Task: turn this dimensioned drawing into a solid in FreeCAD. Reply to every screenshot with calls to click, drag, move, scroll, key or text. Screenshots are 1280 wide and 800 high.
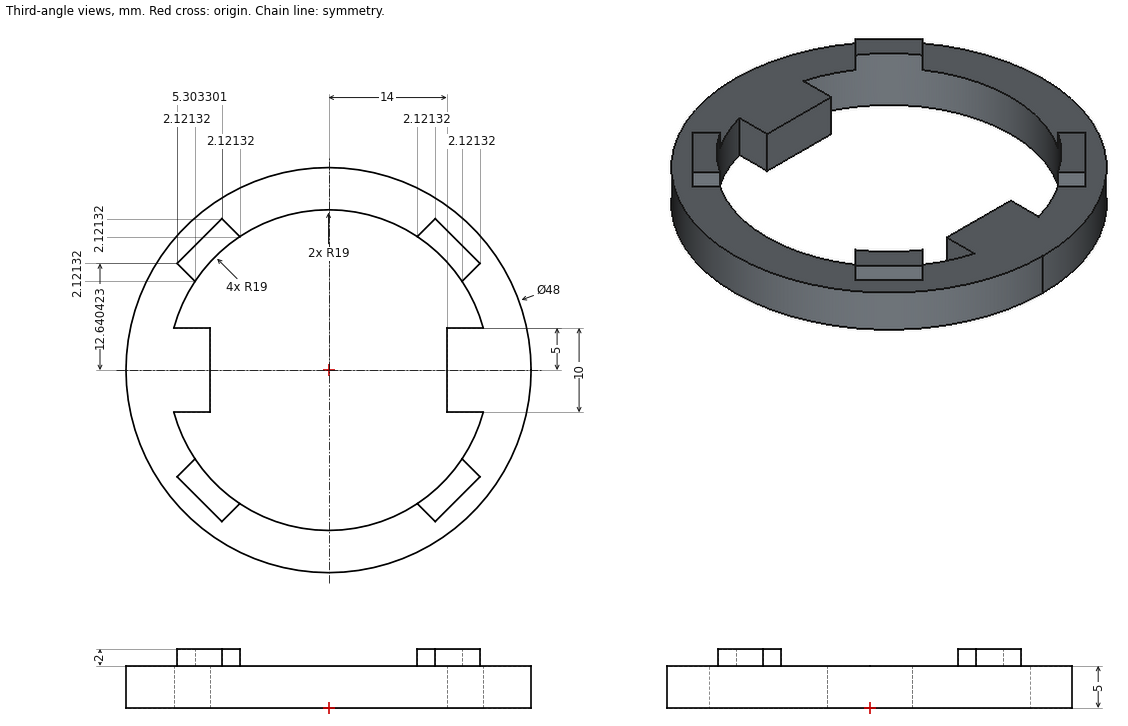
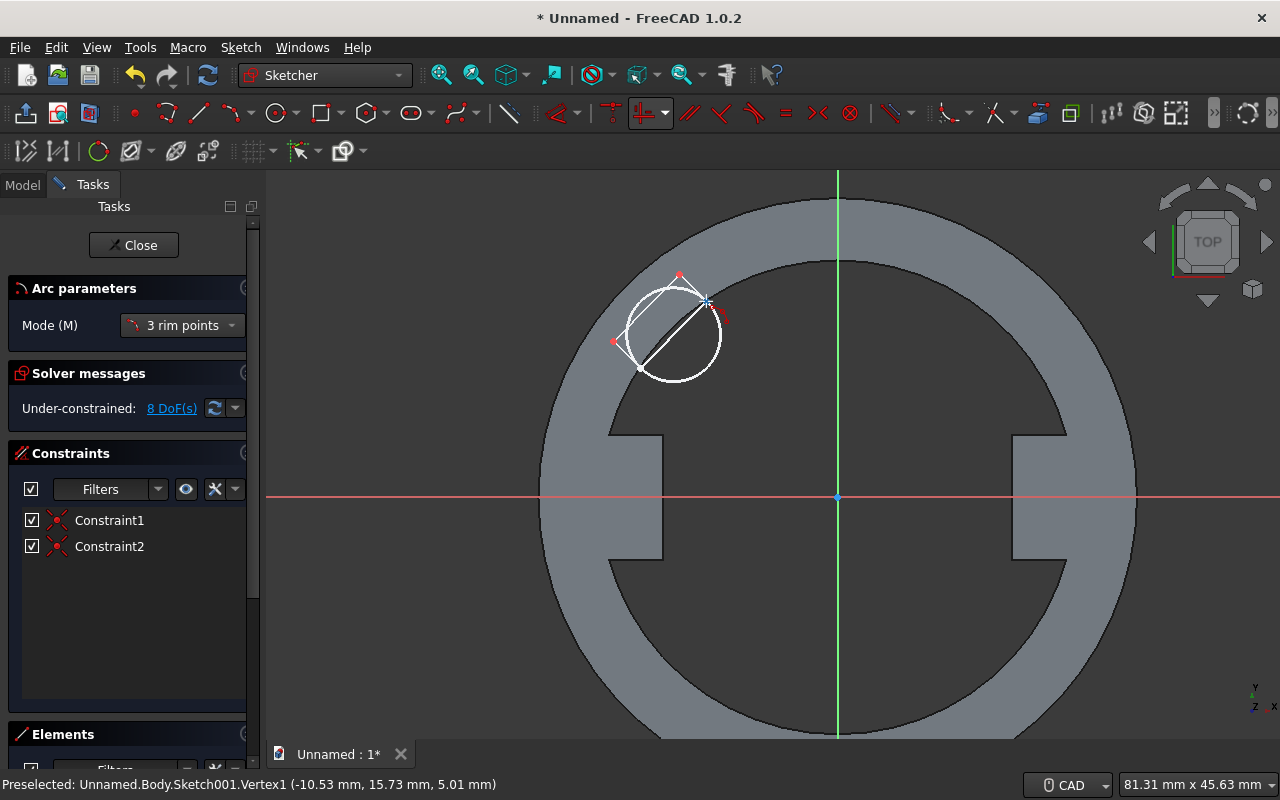
scroll(670, 330, up, 7)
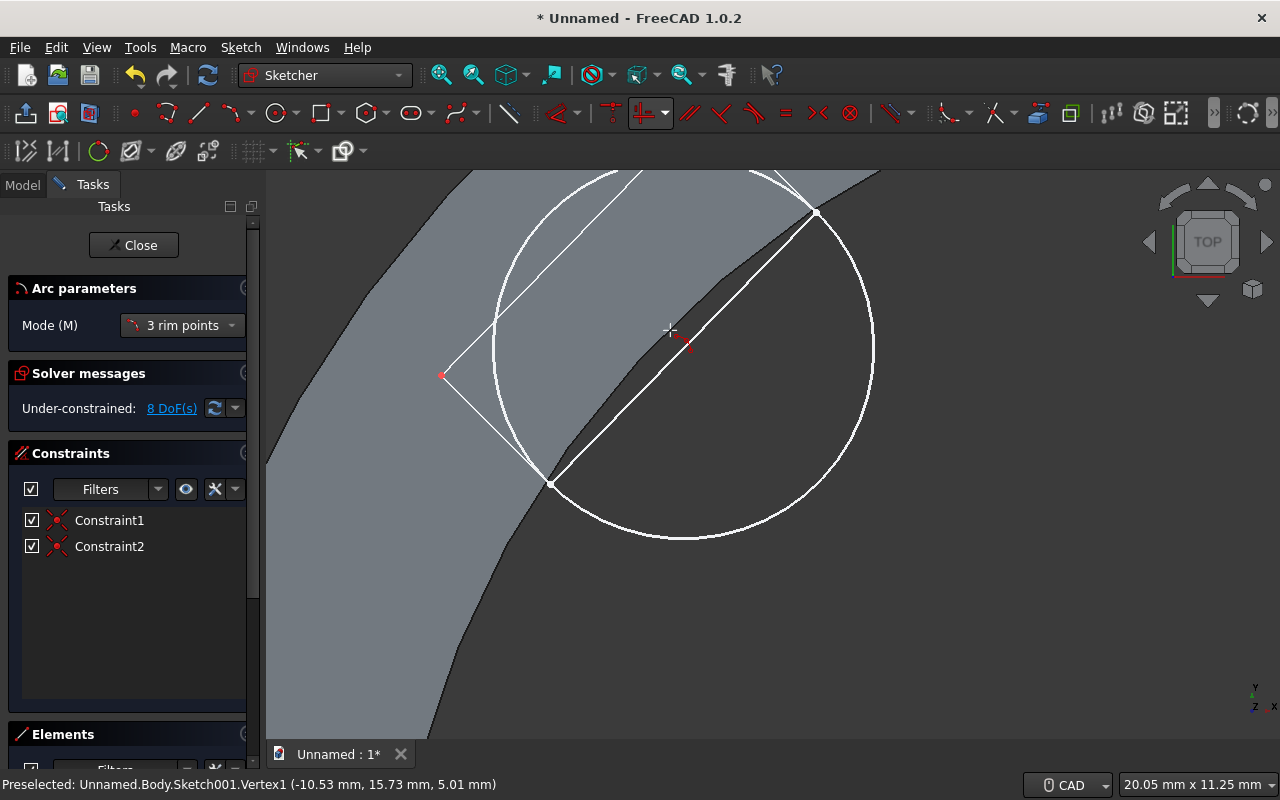
click(670, 328)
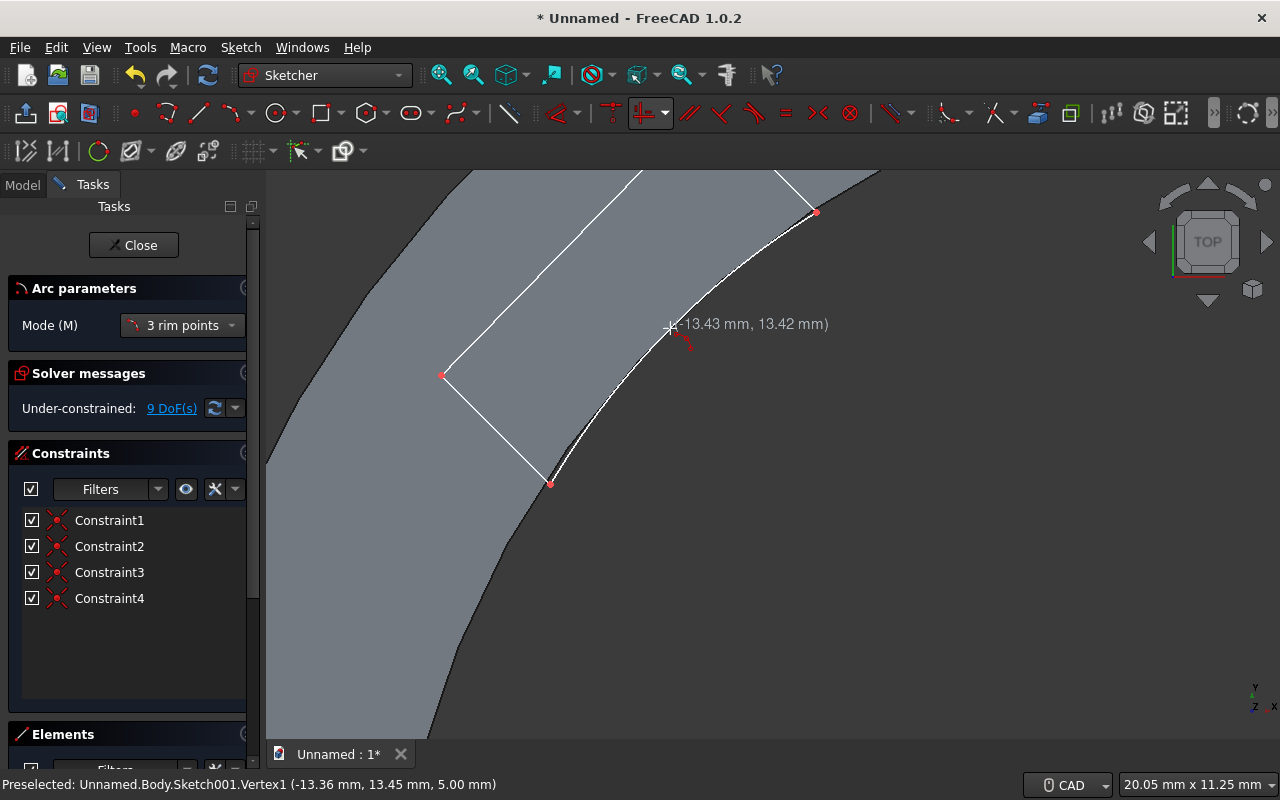
key(g)
key(m)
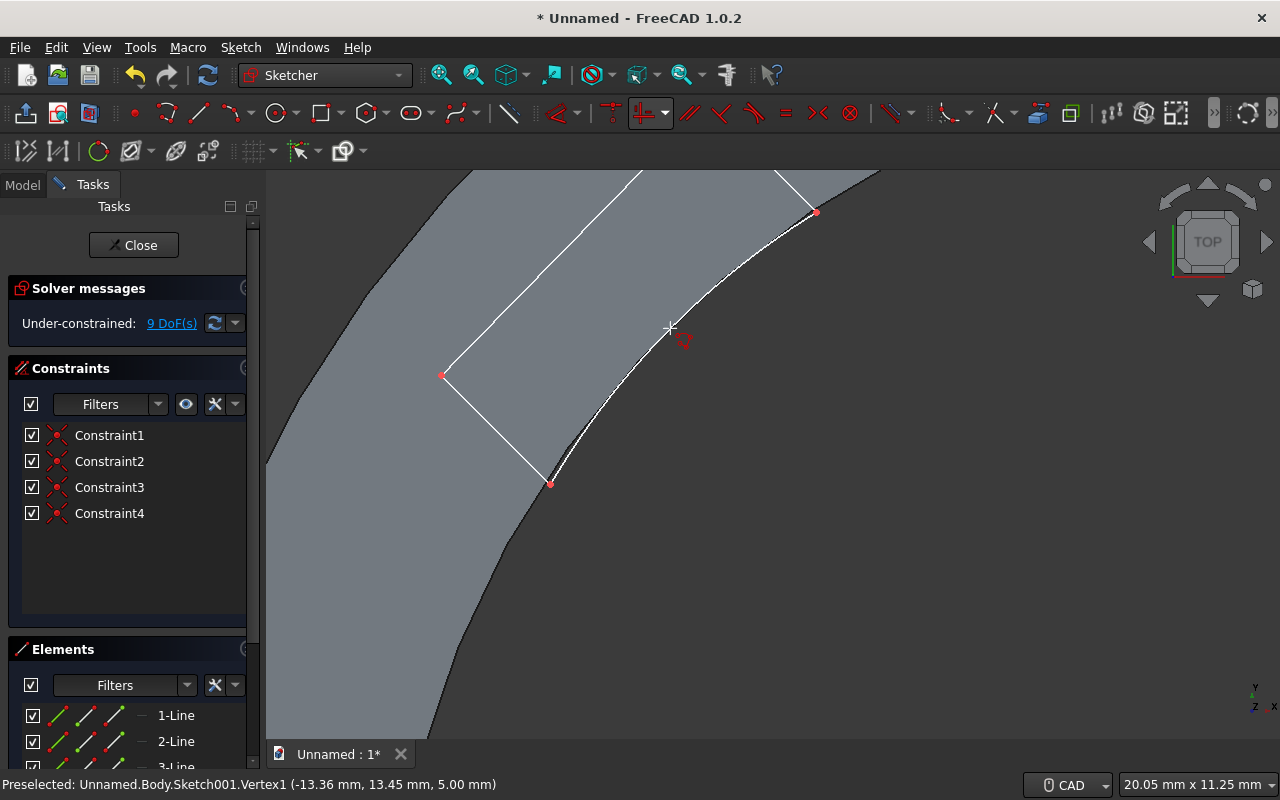
scroll(541, 315, down, 8)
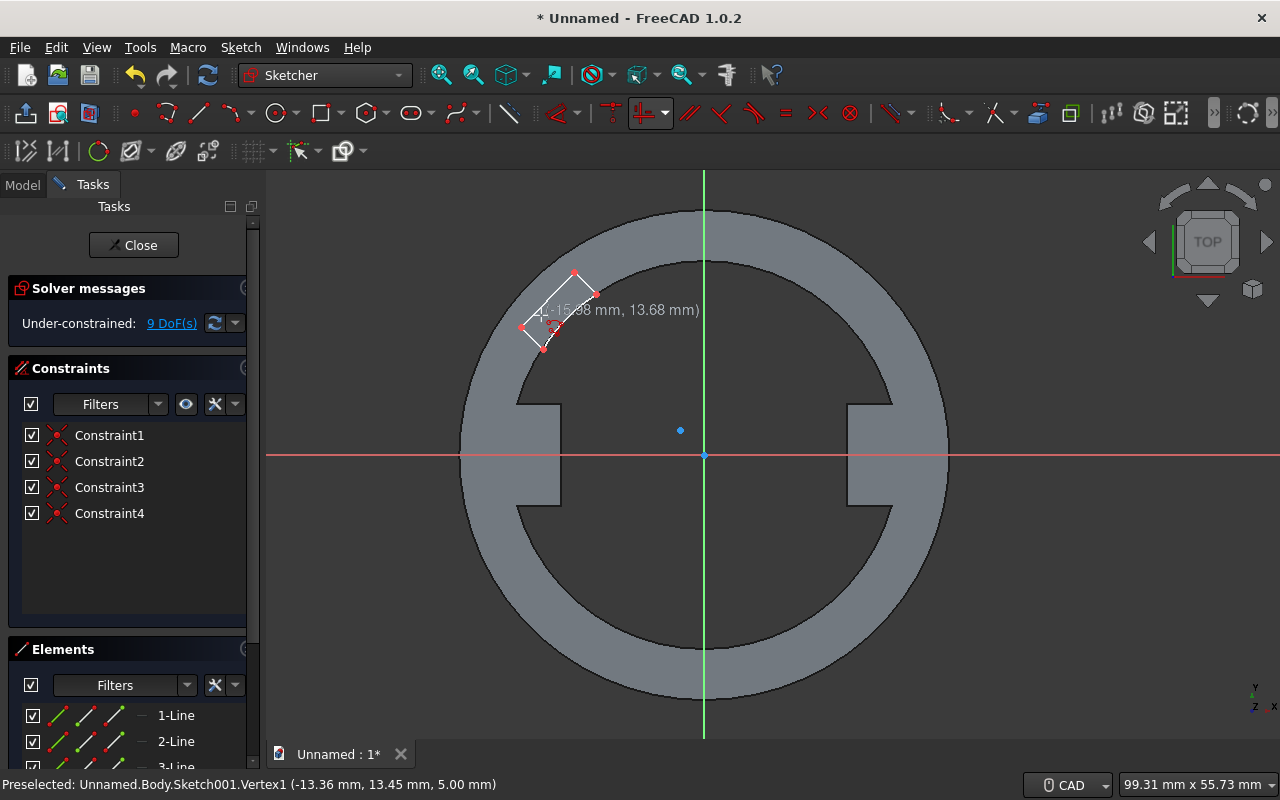
click(866, 348)
click(888, 326)
click(833, 272)
click(812, 294)
right_click(812, 294)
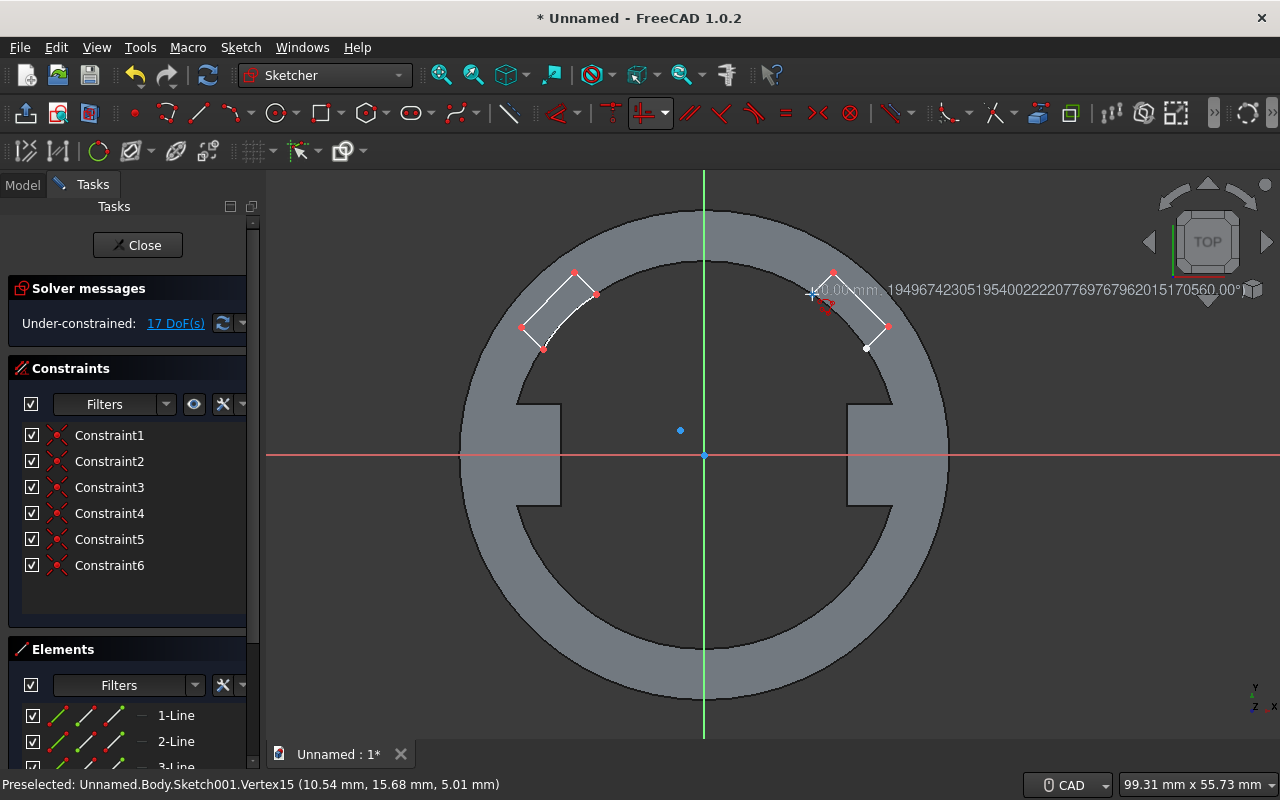
key(g)
key(3)
key(a)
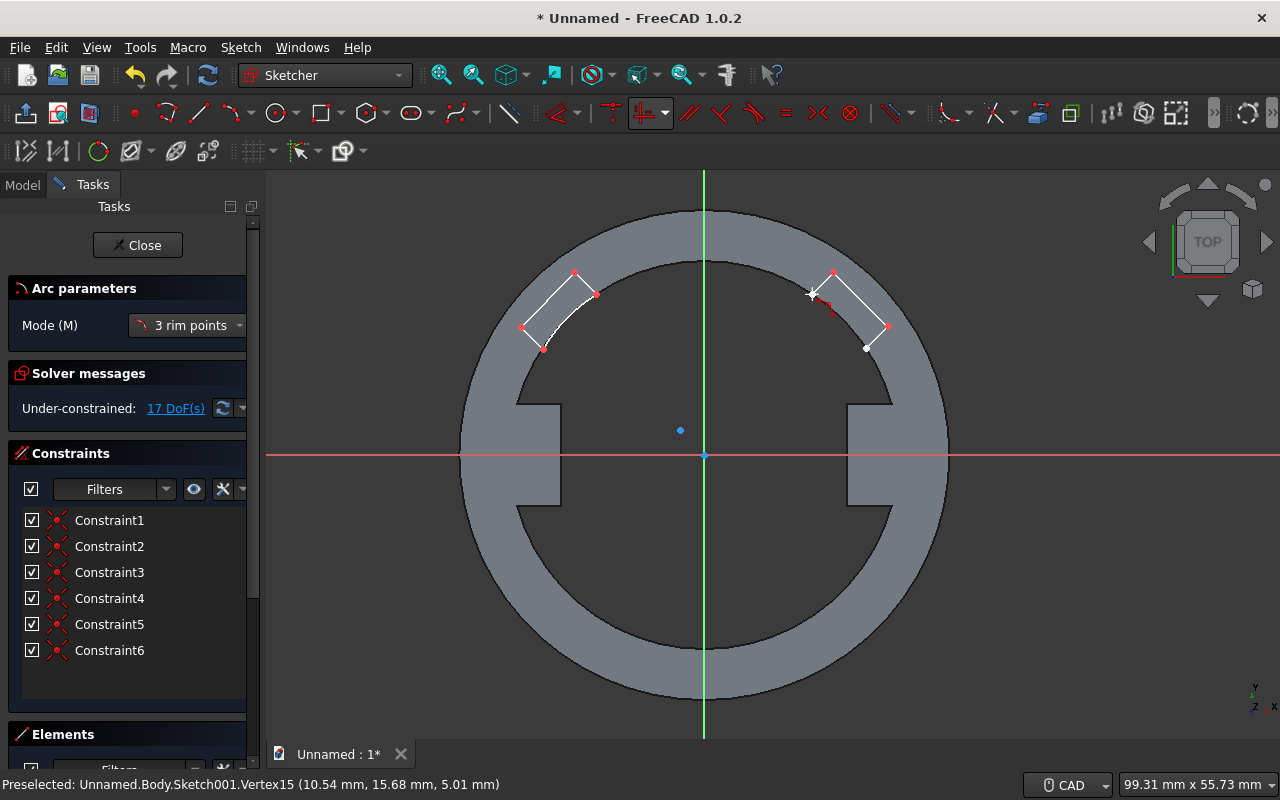
click(812, 295)
click(866, 349)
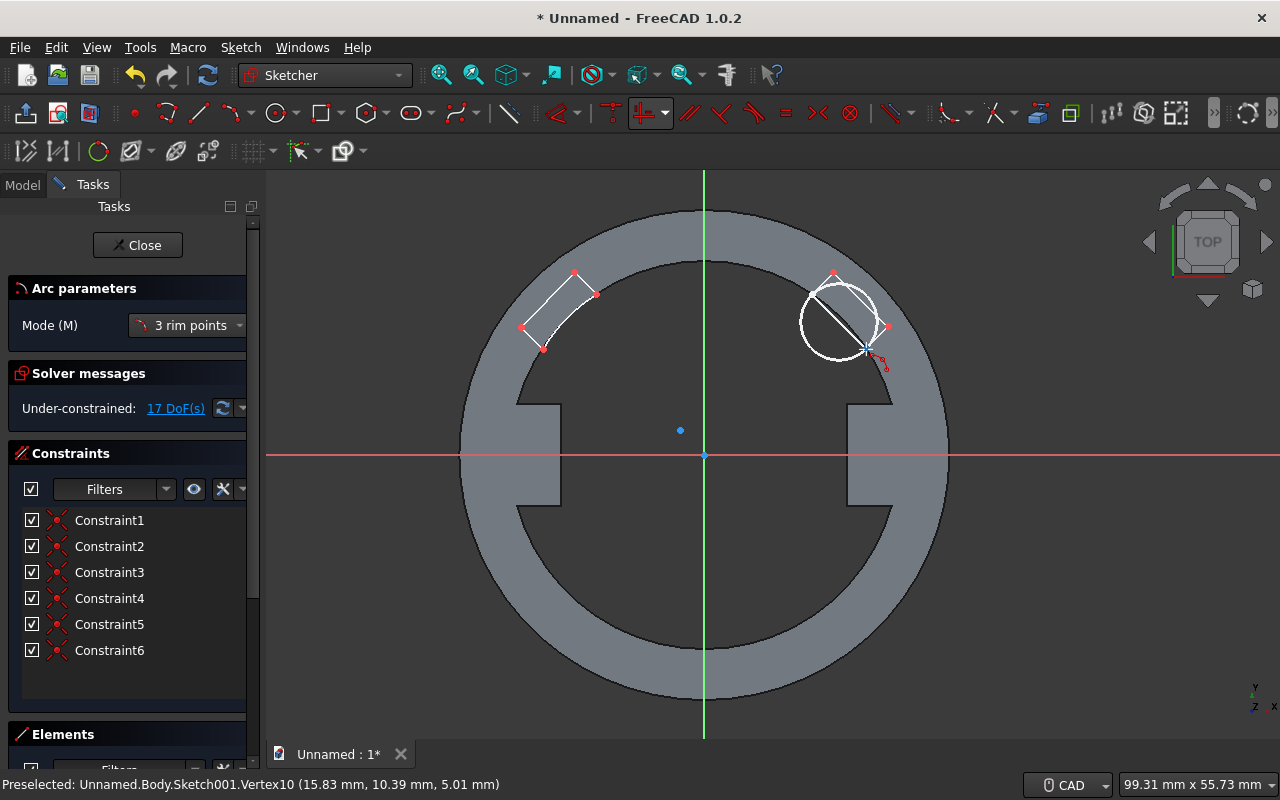
scroll(842, 318, up, 8)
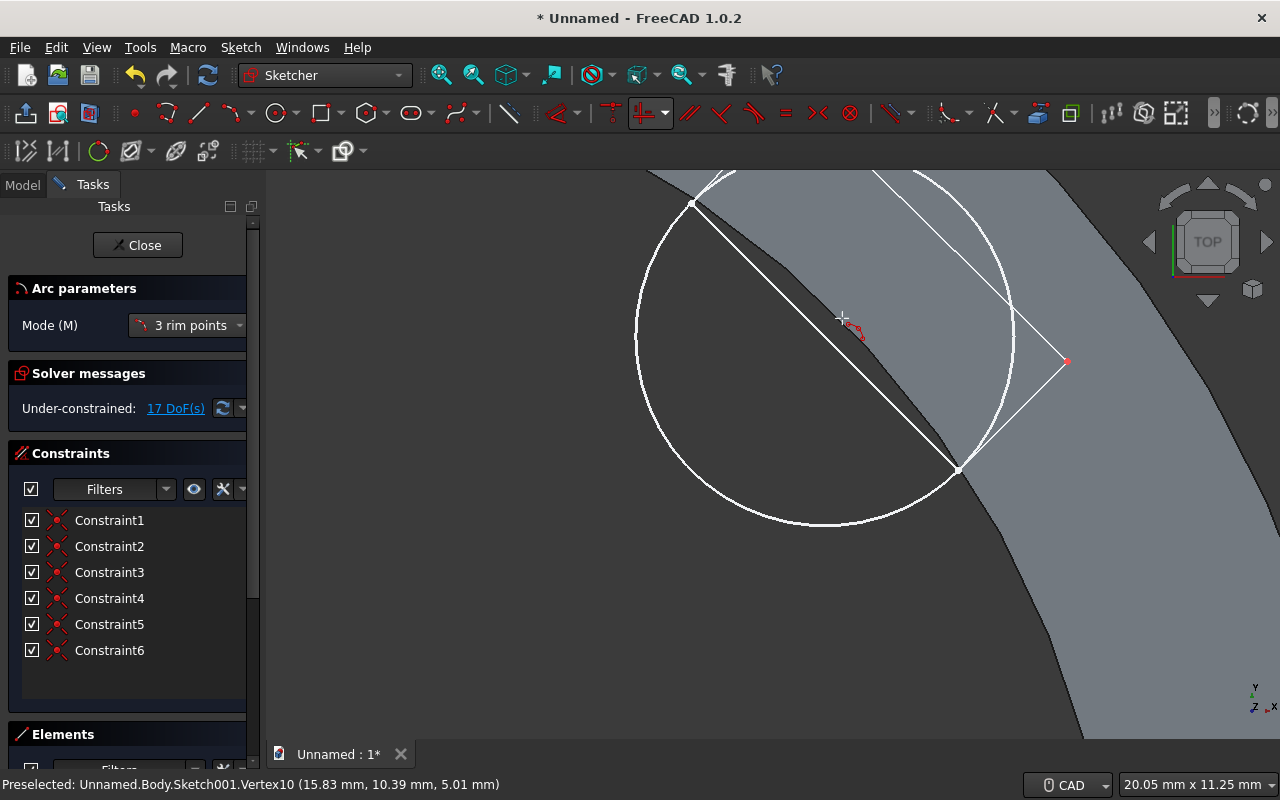
click(837, 317)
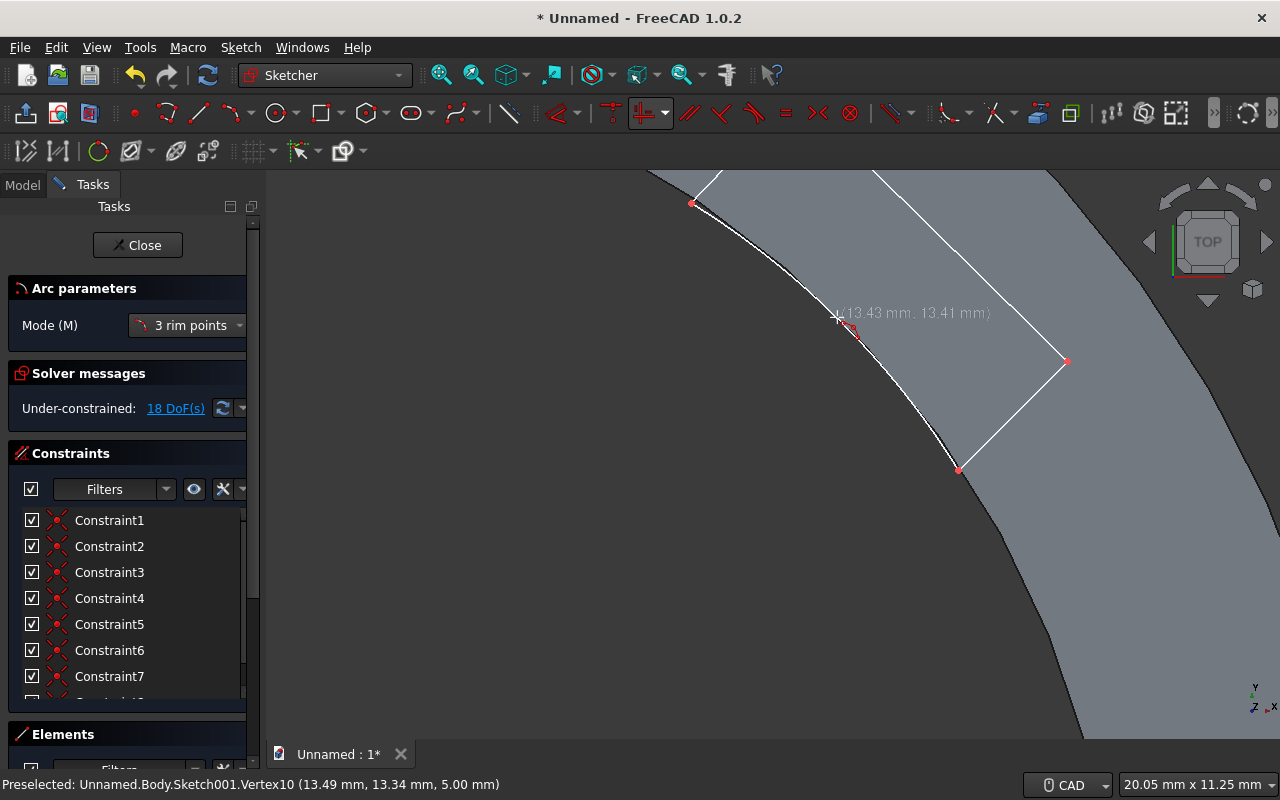
key(g)
key(m)